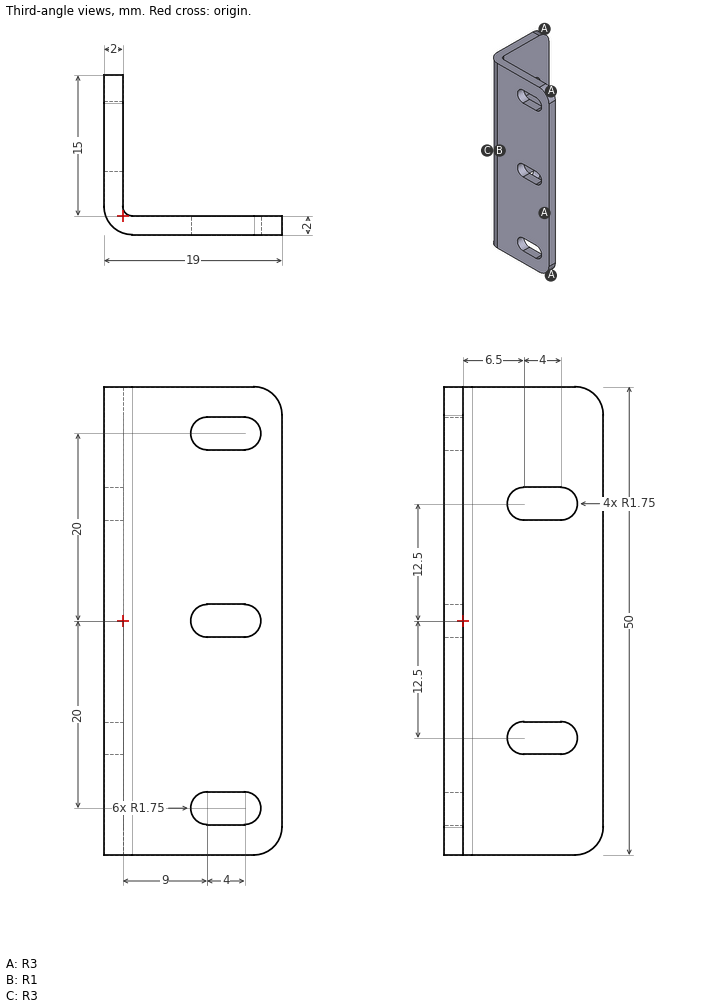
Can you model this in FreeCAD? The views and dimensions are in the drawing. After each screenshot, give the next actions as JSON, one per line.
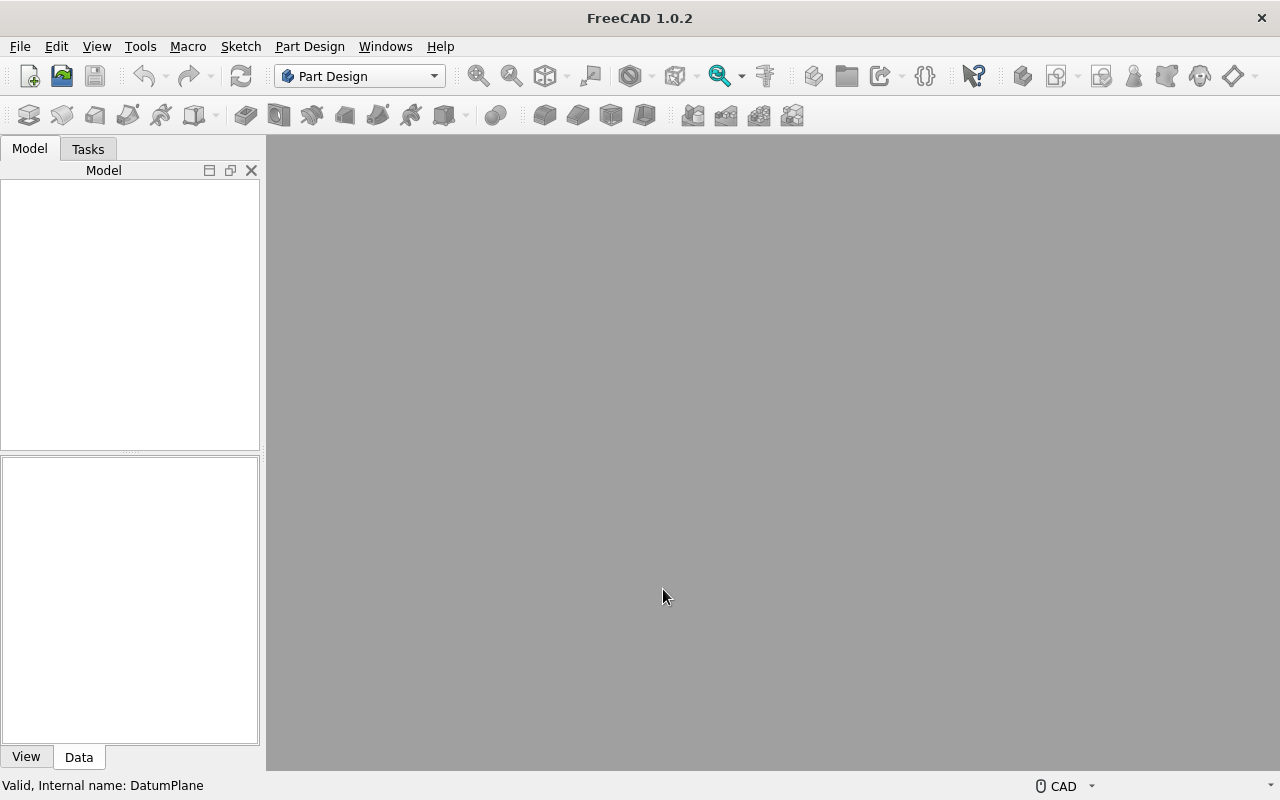
{"action": "left_click", "coordinate": [29, 76]}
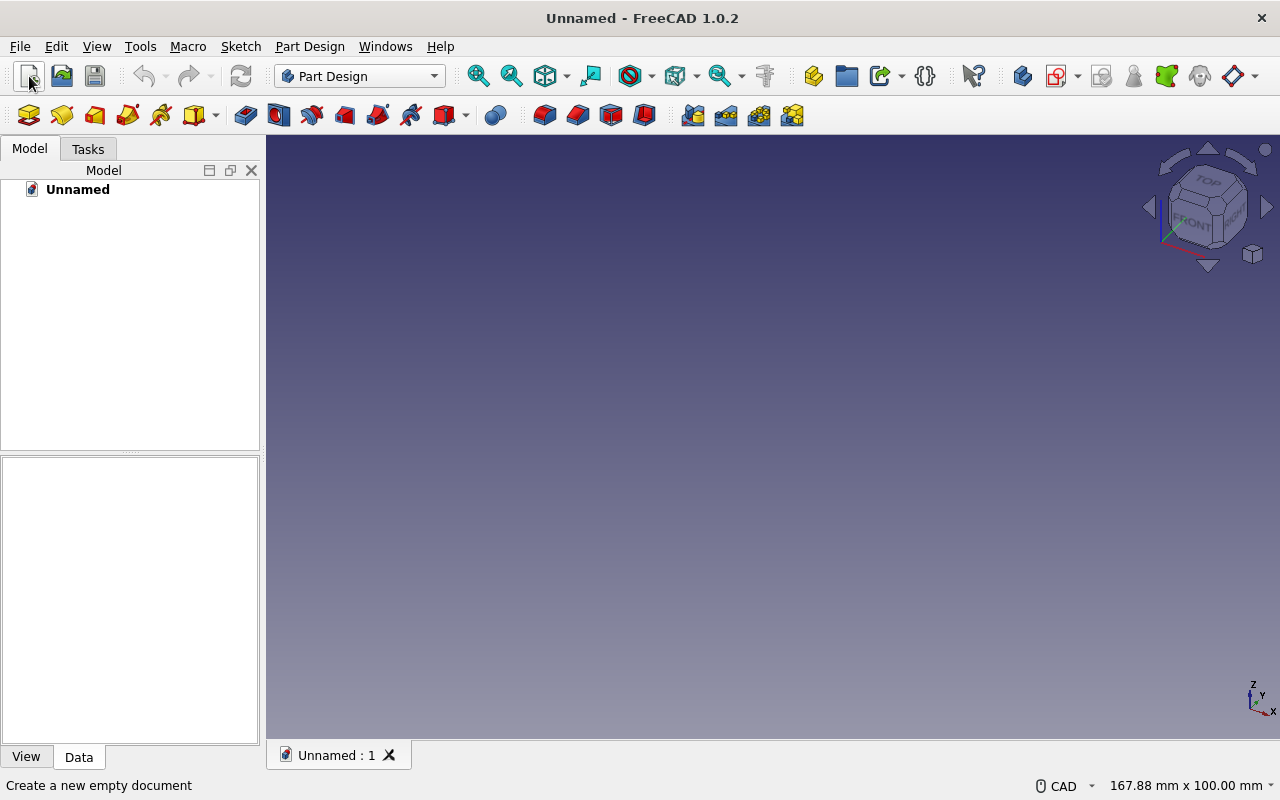
{"action": "left_click", "coordinate": [1056, 76]}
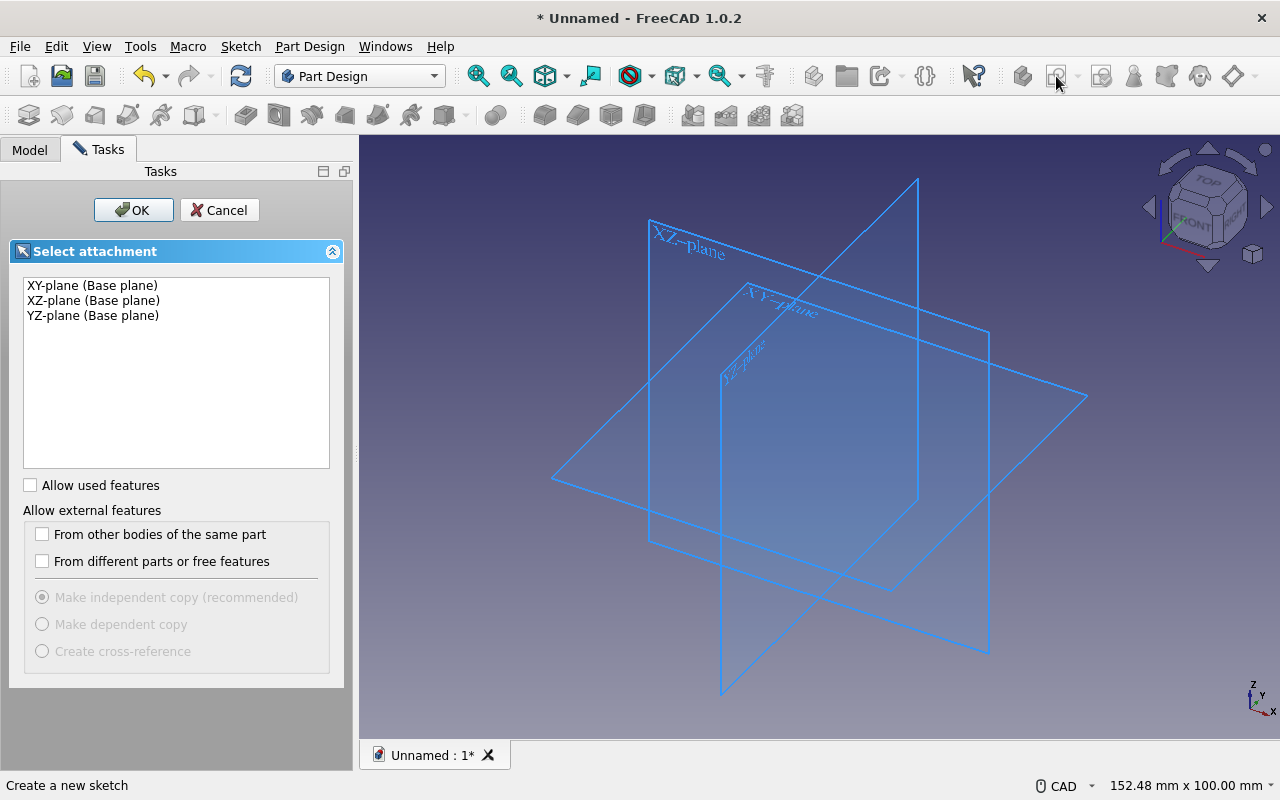
{"action": "left_click", "coordinate": [84, 286]}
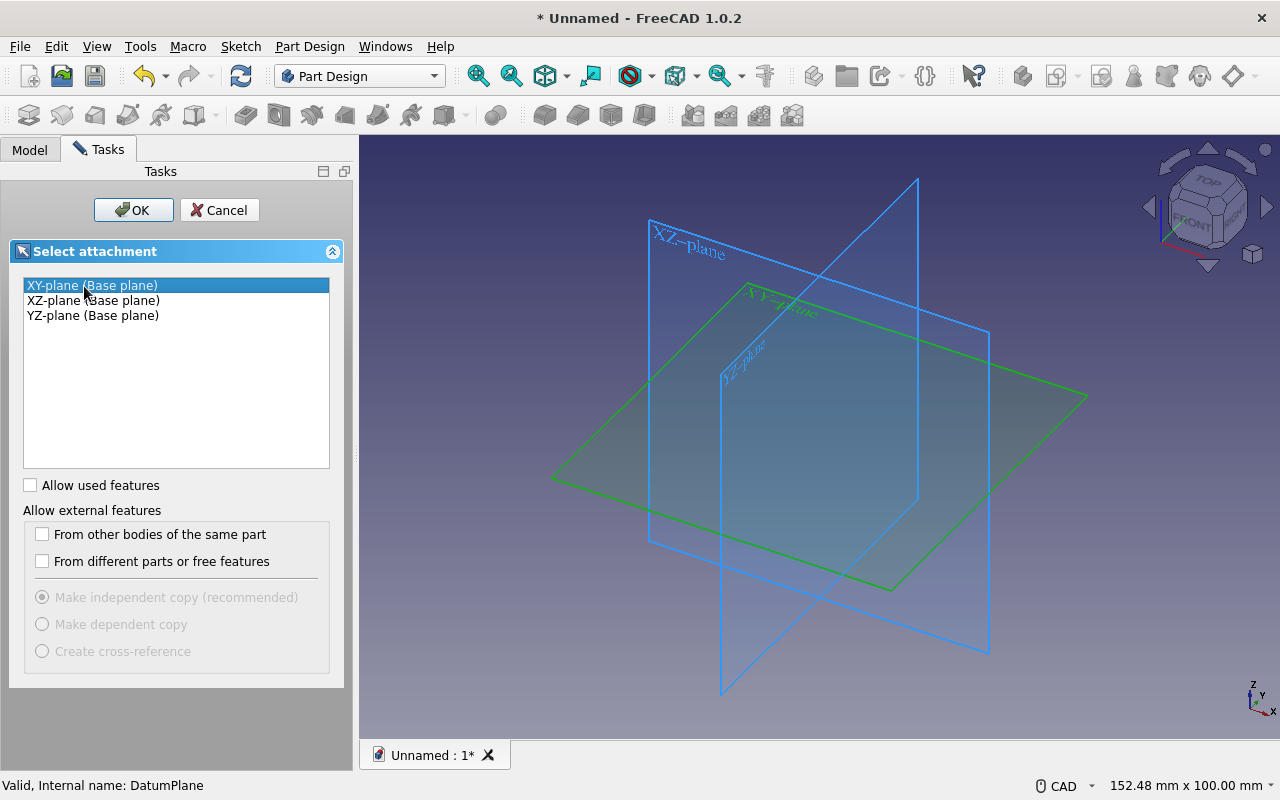
{"action": "left_click", "coordinate": [134, 210]}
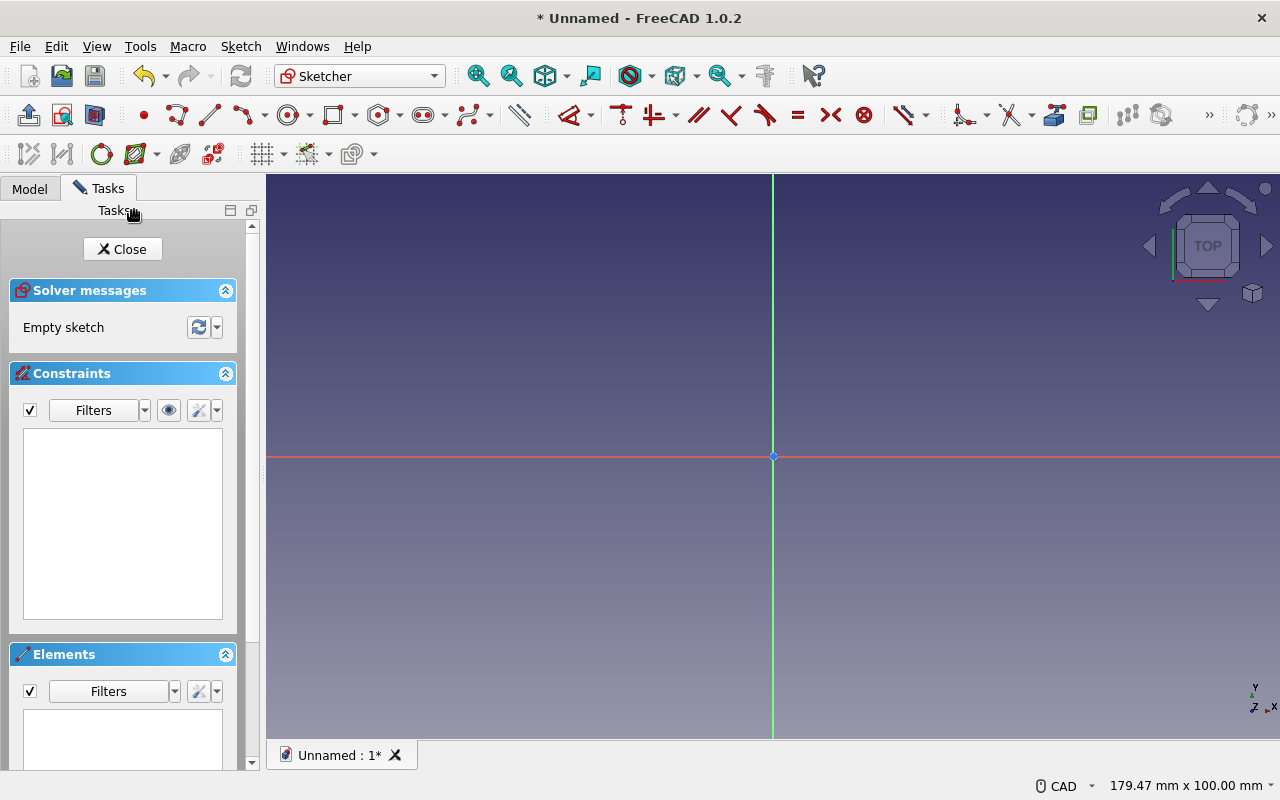
{"action": "scroll", "coordinate": [852, 408], "scroll_direction": "up", "scroll_amount": 7}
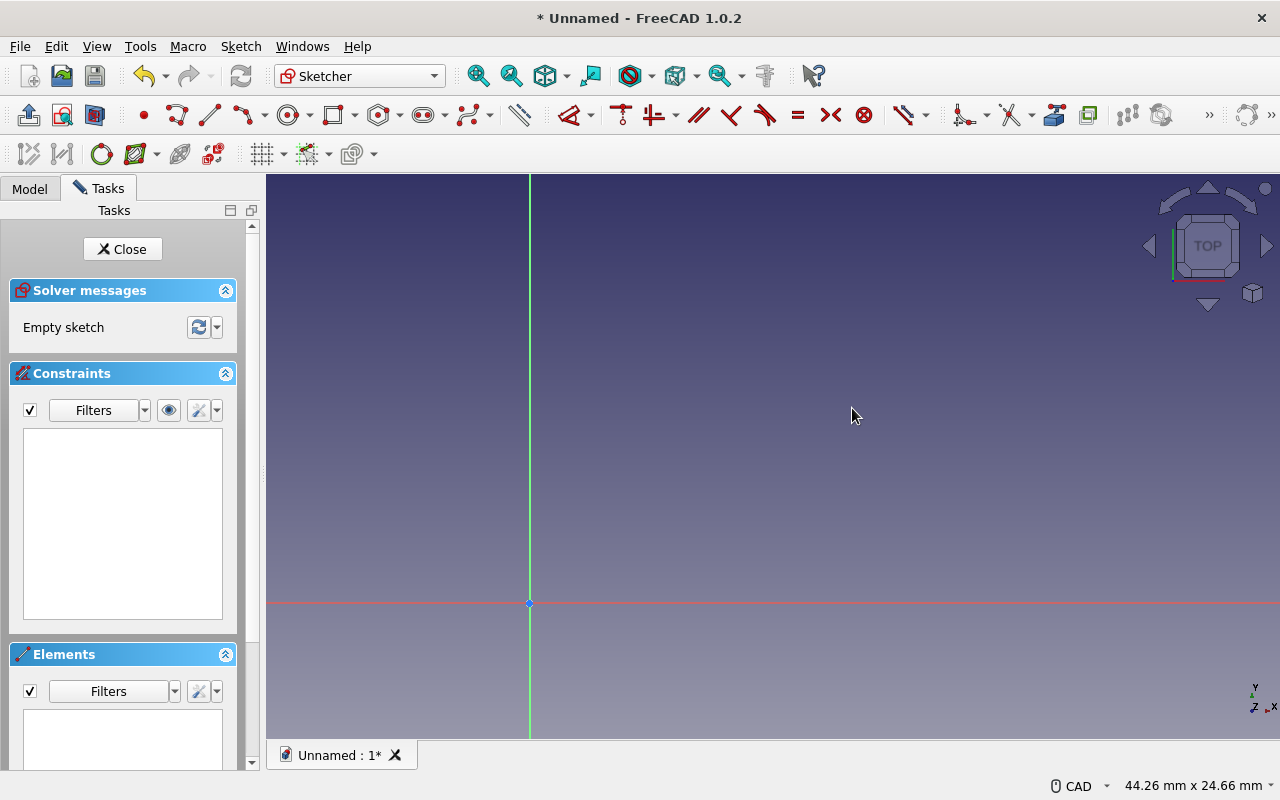
{"action": "left_click", "coordinate": [177, 116]}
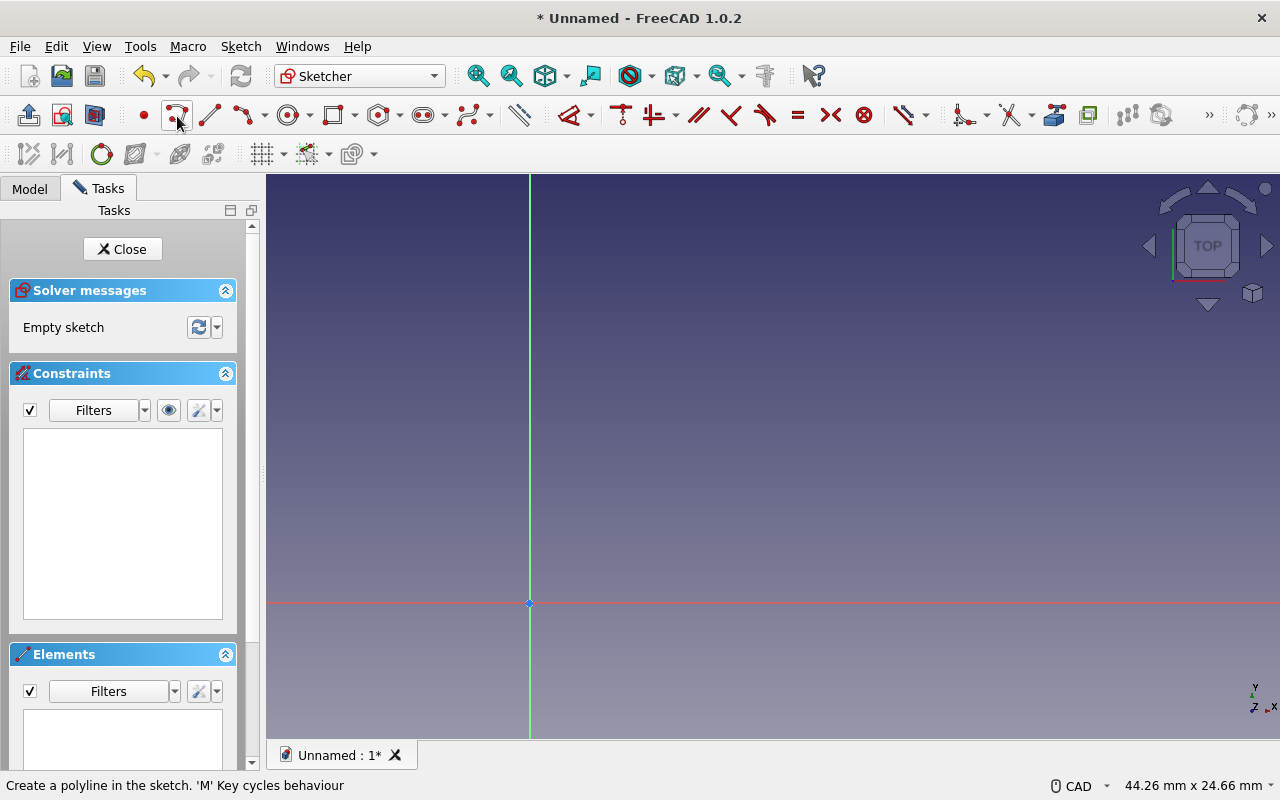
{"action": "left_click", "coordinate": [530, 603]}
{"action": "left_click", "coordinate": [539, 260]}
{"action": "left_click", "coordinate": [484, 260]}
{"action": "left_click", "coordinate": [484, 649]}
{"action": "left_click", "coordinate": [919, 649]}
{"action": "left_click", "coordinate": [919, 594]}
{"action": "left_click", "coordinate": [530, 603]}
{"action": "key", "text": "Escape"}
{"action": "key", "text": "Escape"}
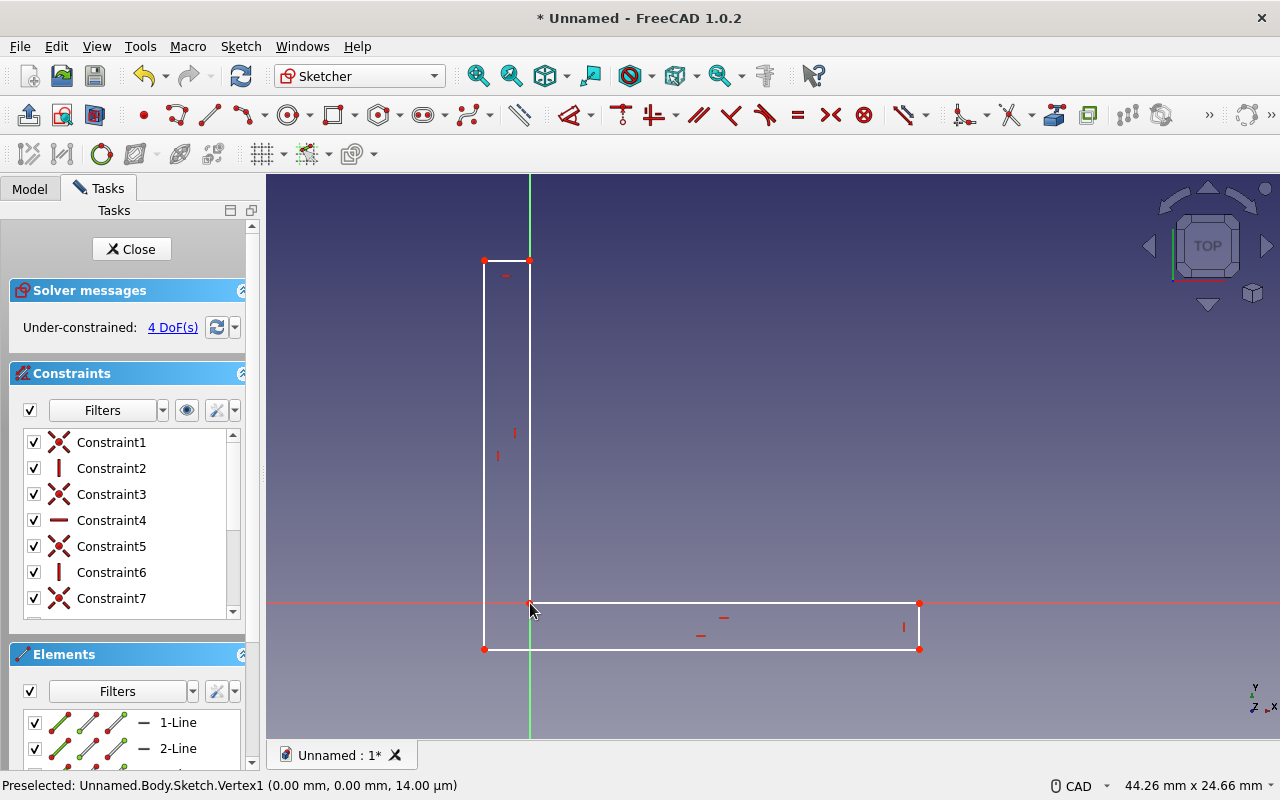
{"action": "left_click", "coordinate": [516, 261]}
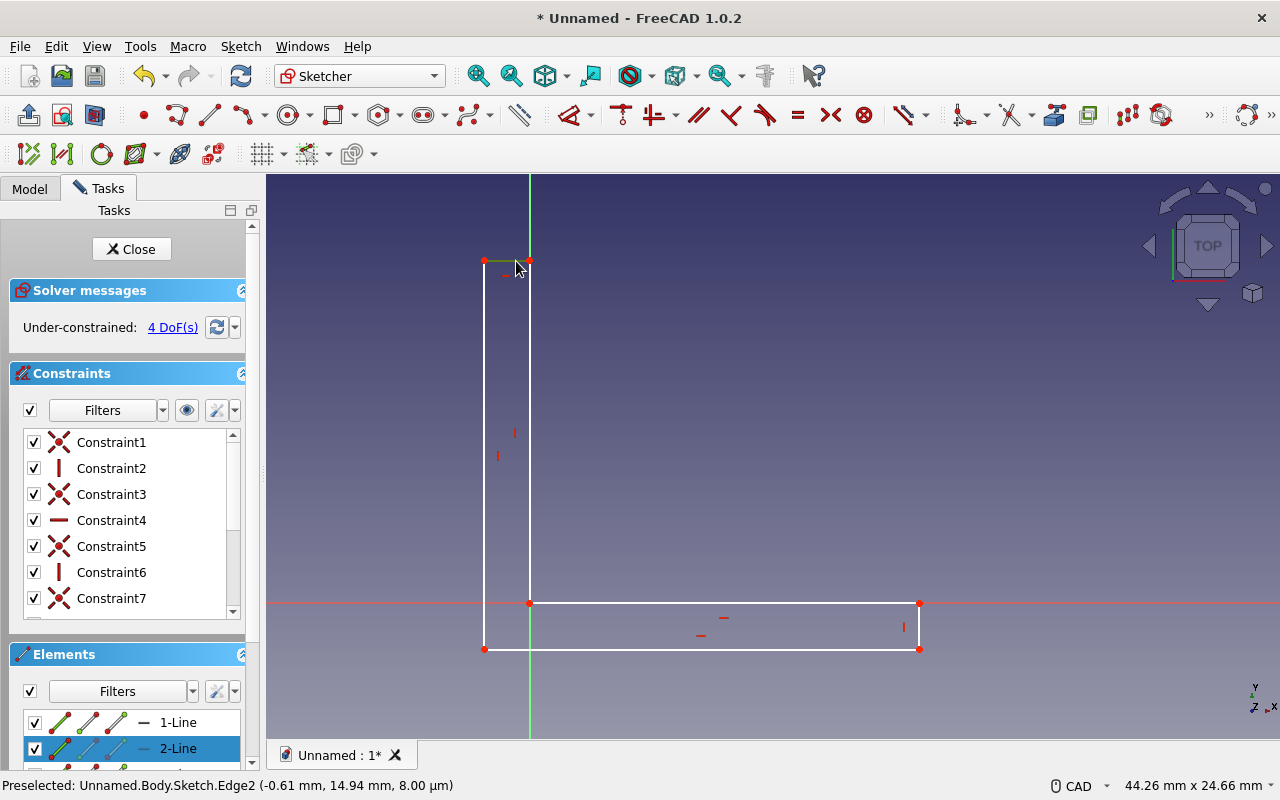
{"action": "key", "text": "l"}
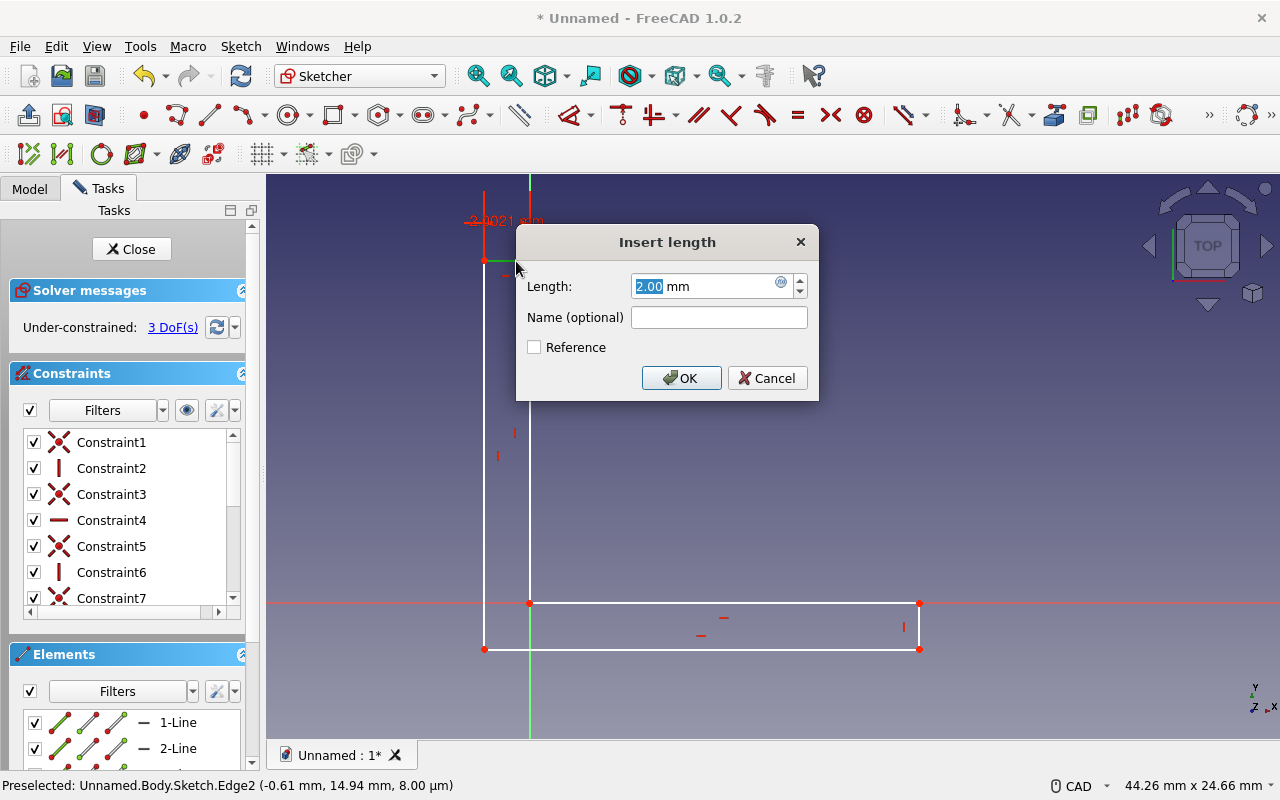
{"action": "type", "text": "2"}
{"action": "key", "text": "Return"}